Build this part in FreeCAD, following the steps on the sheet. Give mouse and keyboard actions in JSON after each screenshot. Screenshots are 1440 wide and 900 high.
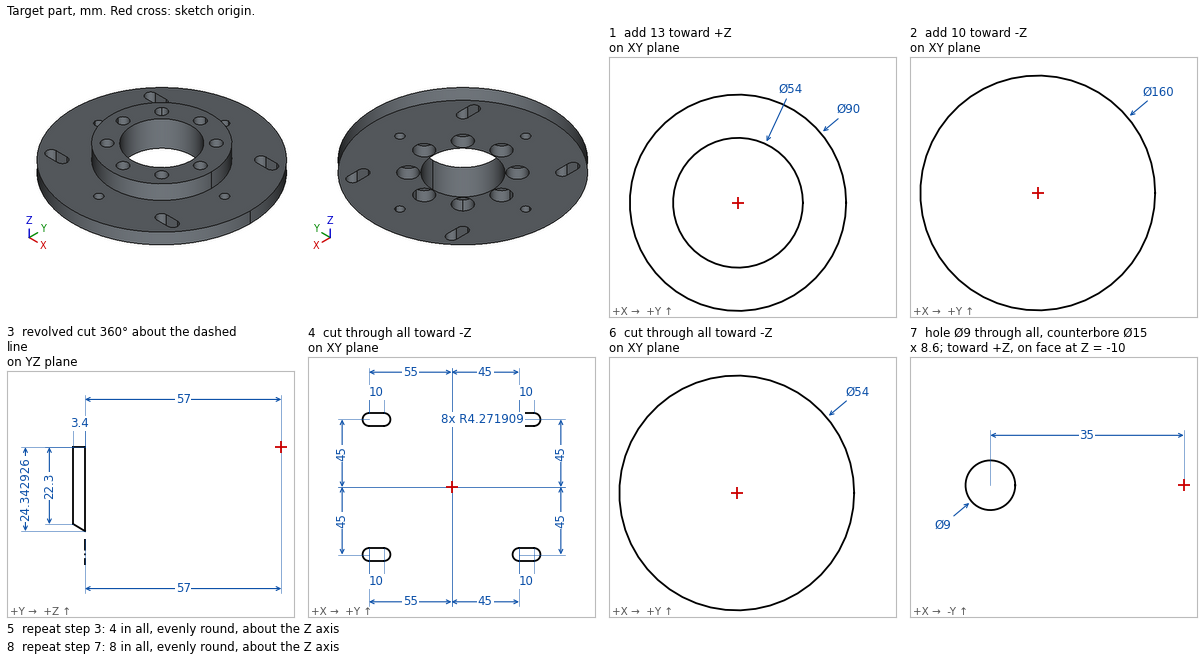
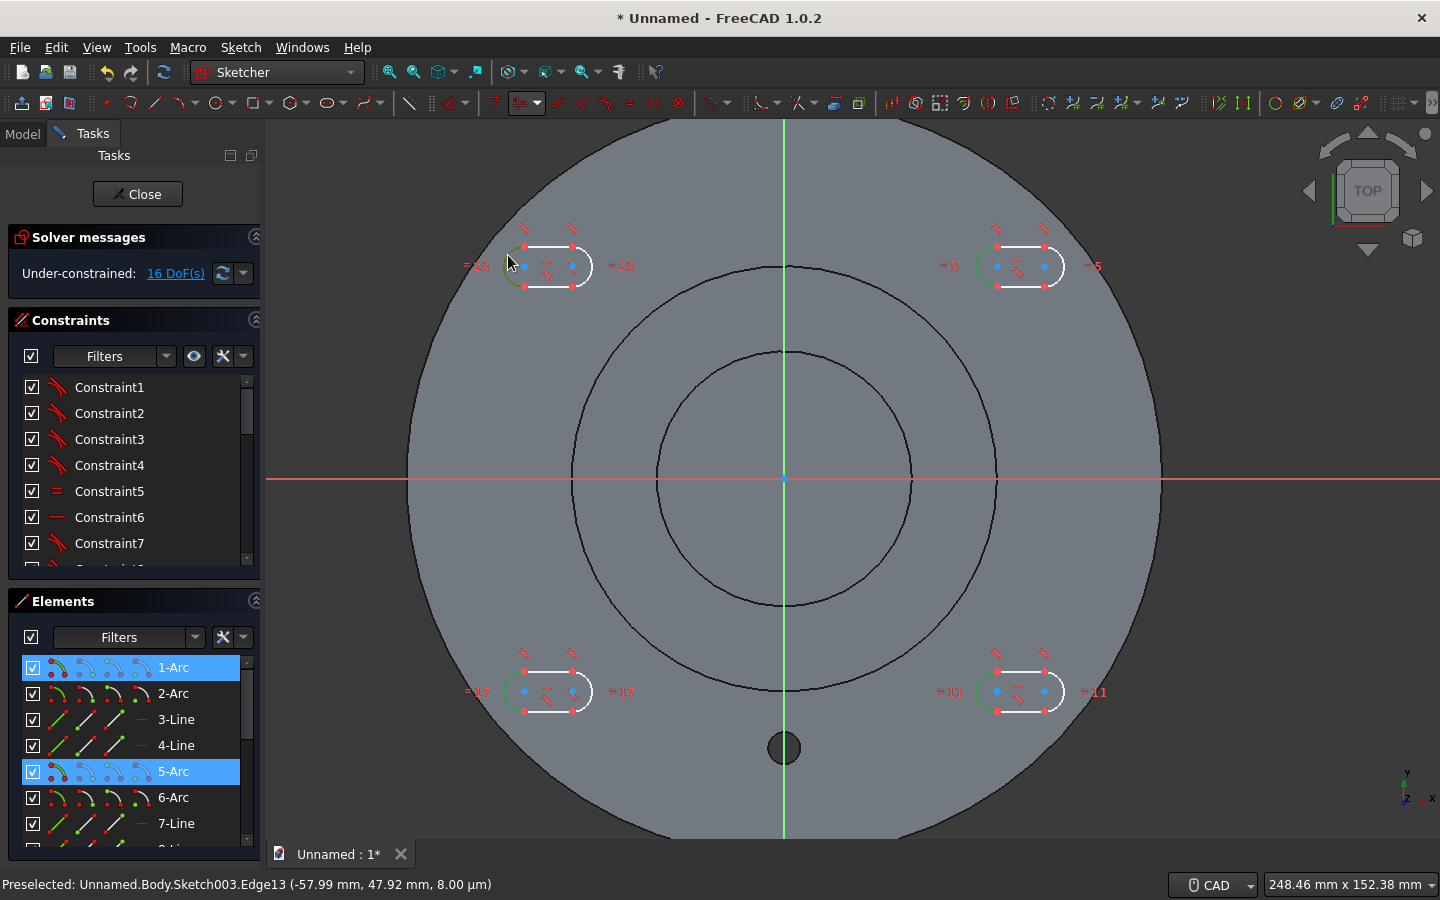
{"action": "key", "text": "e"}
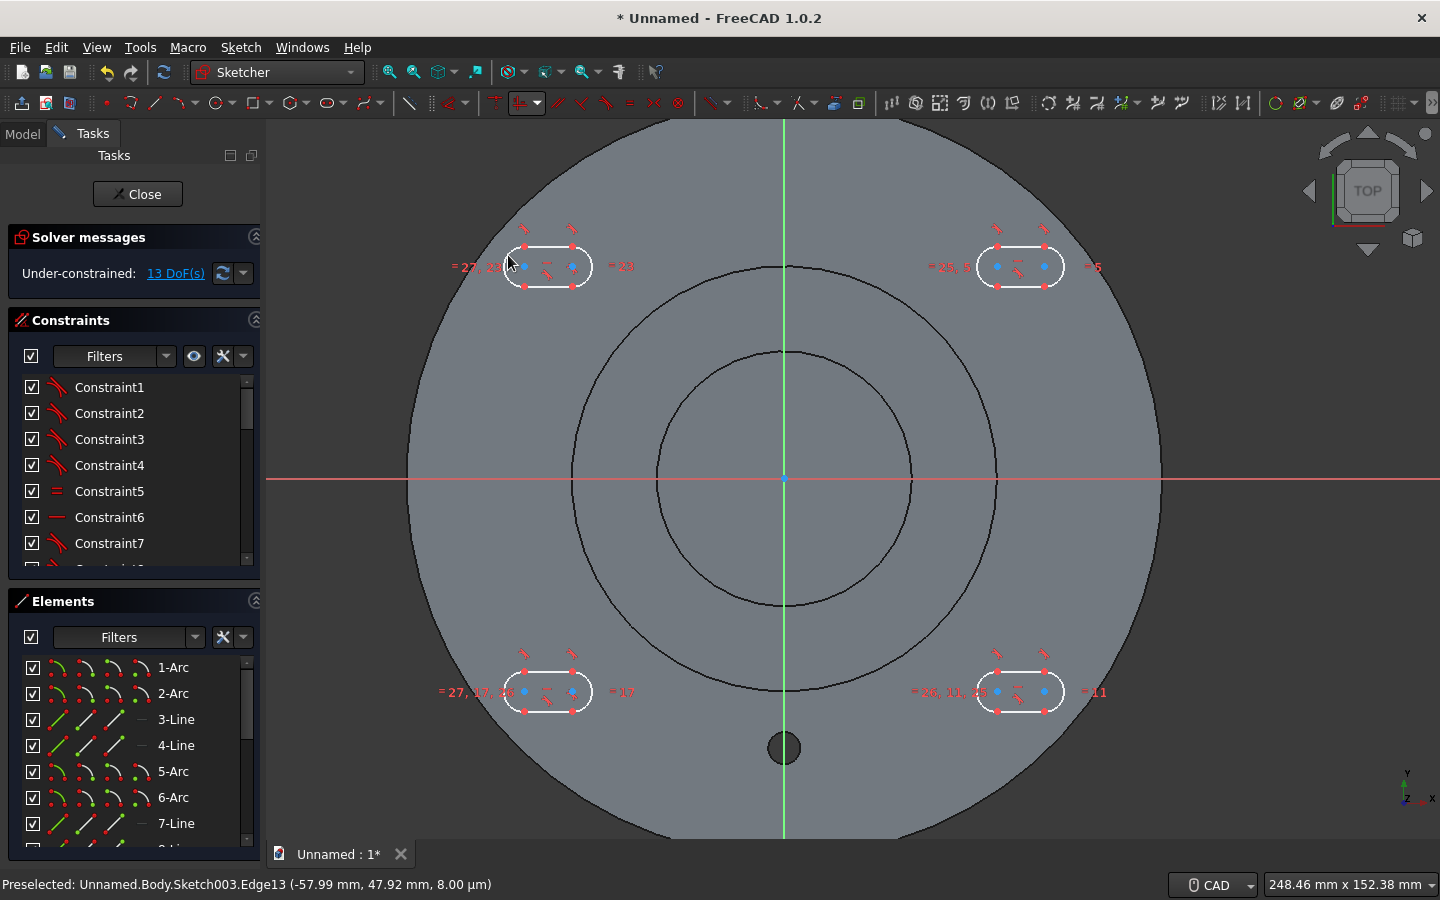
{"action": "key", "text": "d"}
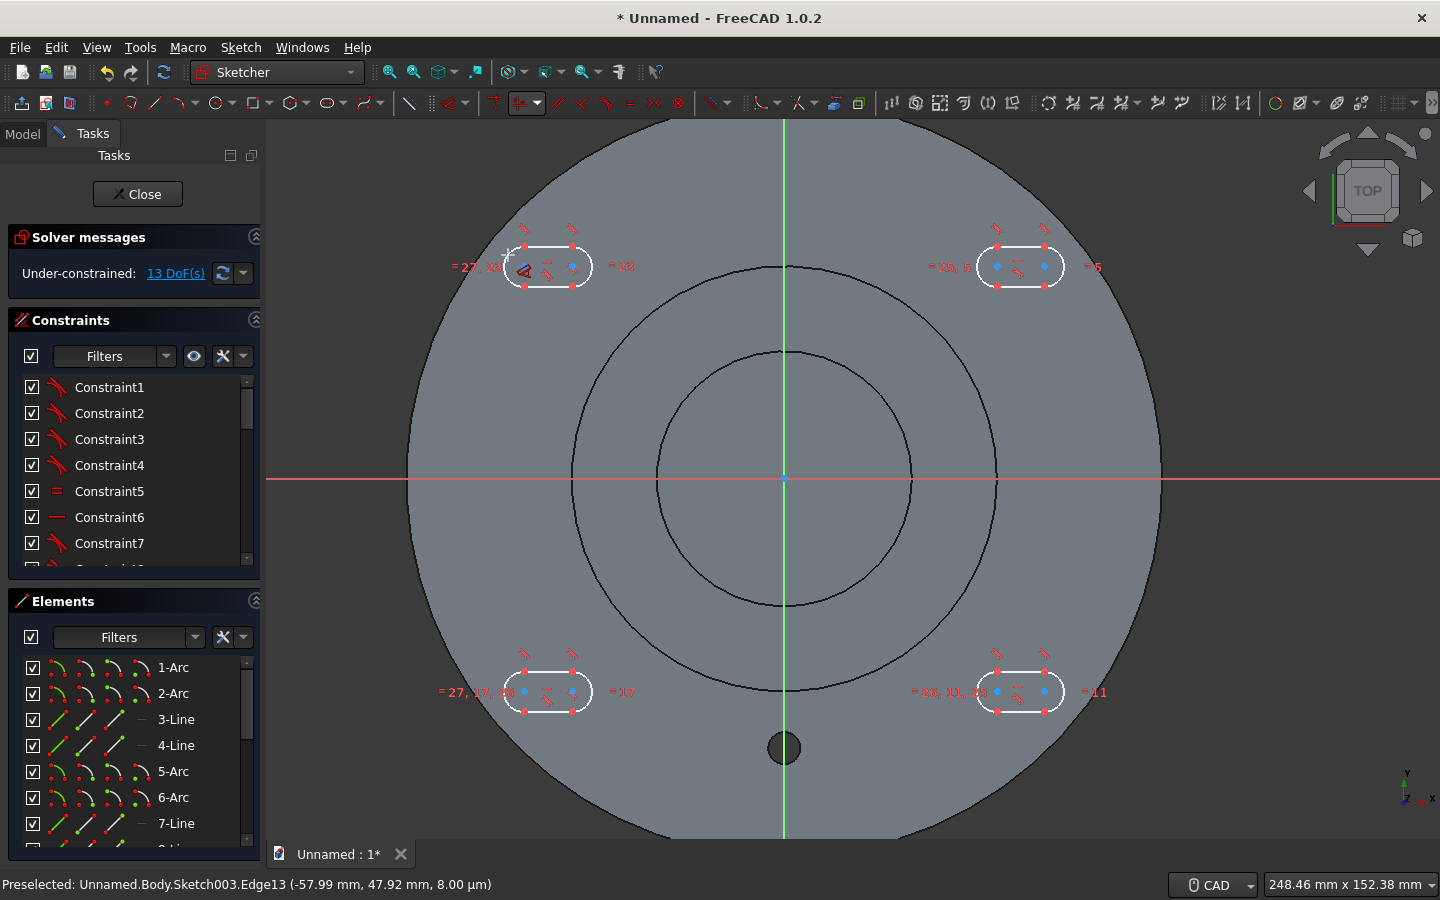
{"action": "scroll", "coordinate": [981, 255], "scroll_direction": "up", "scroll_amount": 4}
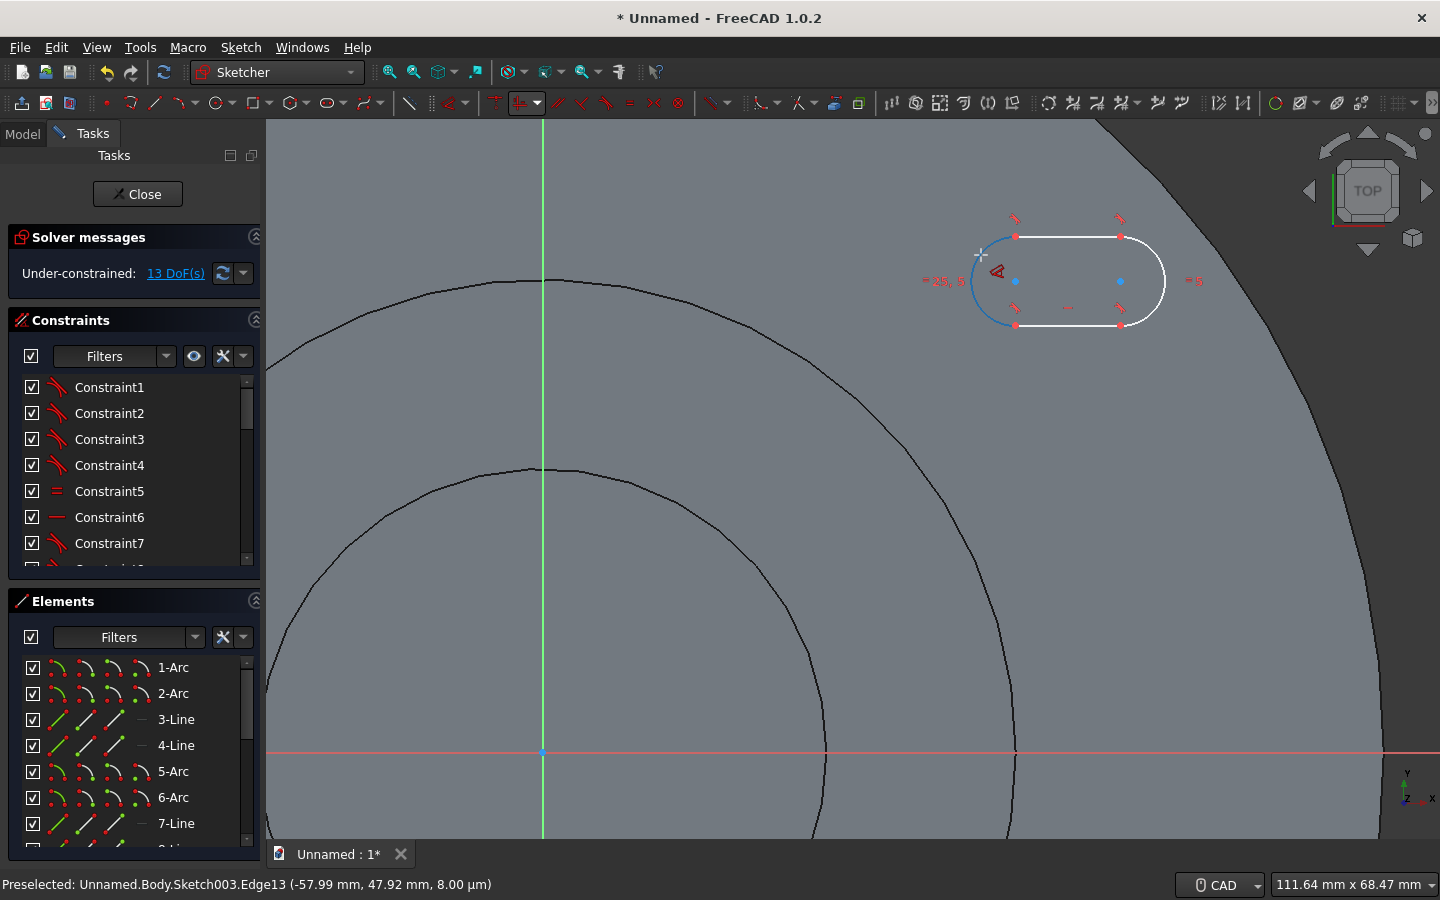
{"action": "left_click", "coordinate": [980, 255]}
{"action": "left_click", "coordinate": [954, 236]}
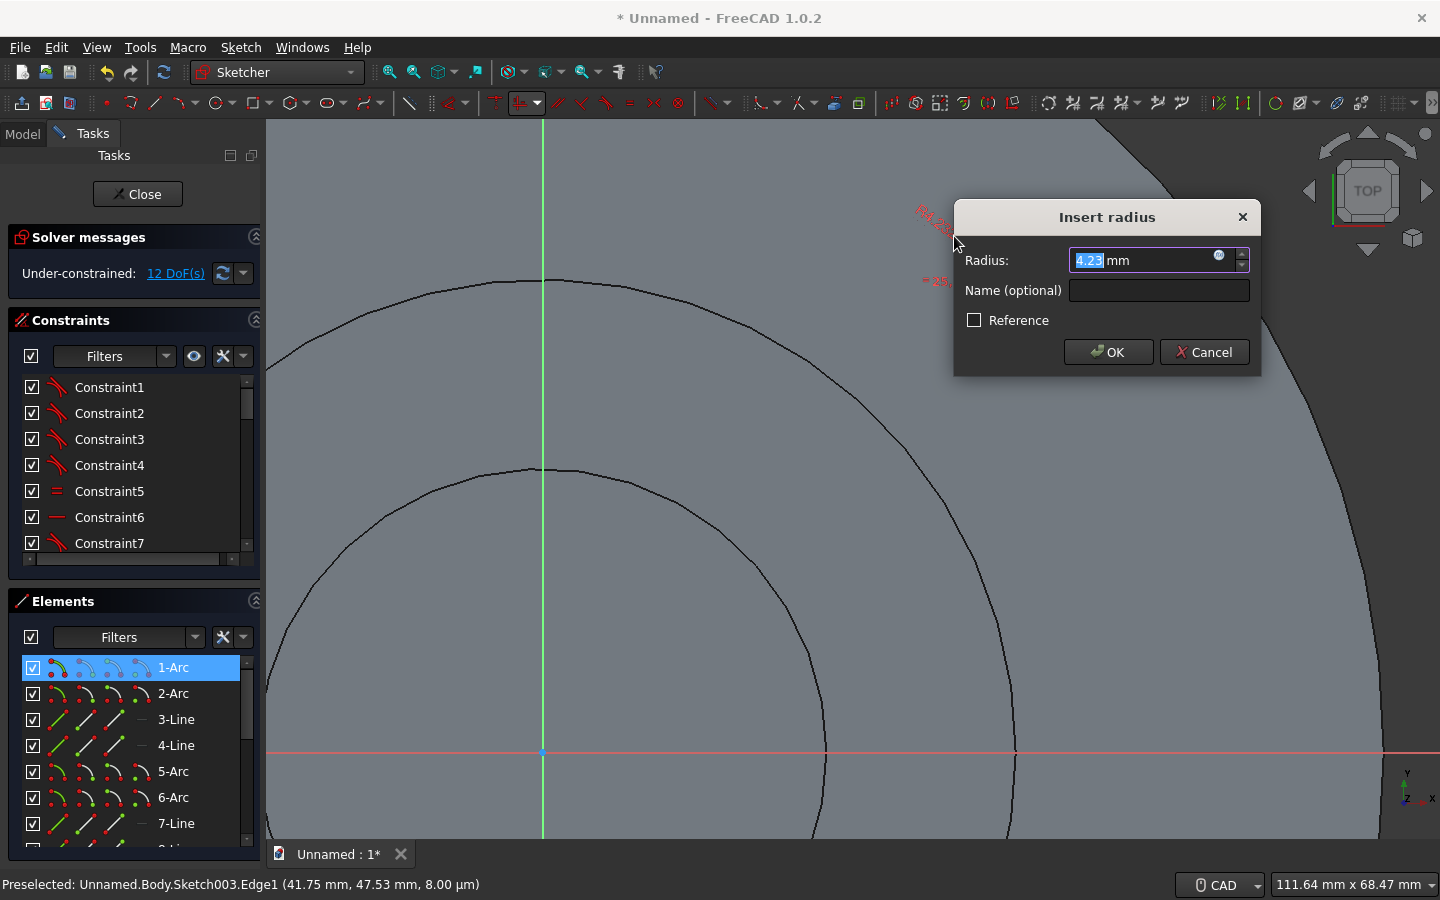
{"action": "type", "text": "4.271909"}
{"action": "key", "text": "Return"}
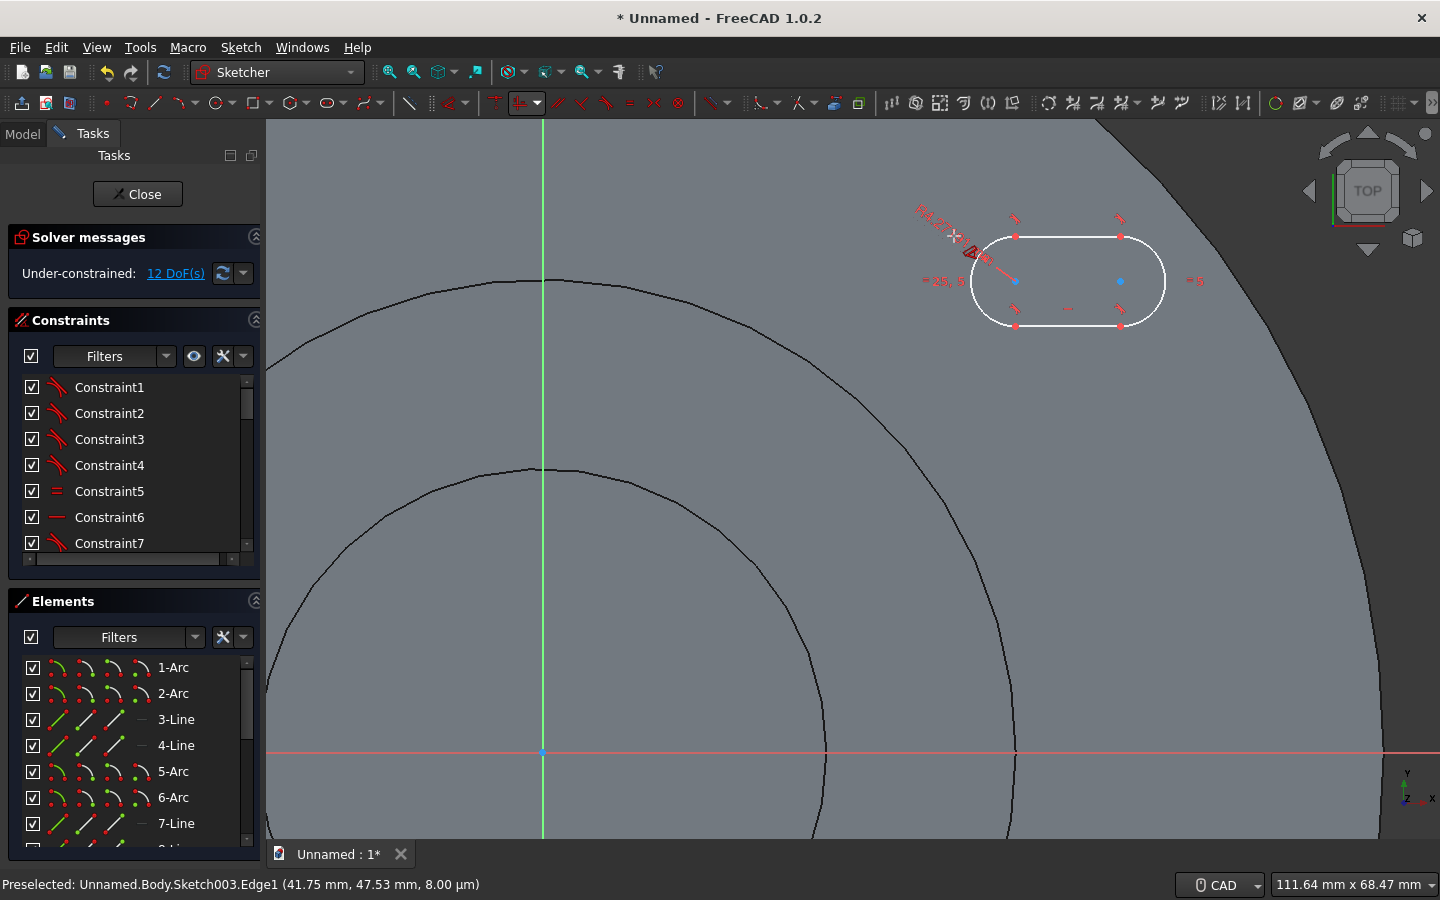
{"action": "left_click", "coordinate": [1047, 237]}
{"action": "left_click", "coordinate": [1068, 203]}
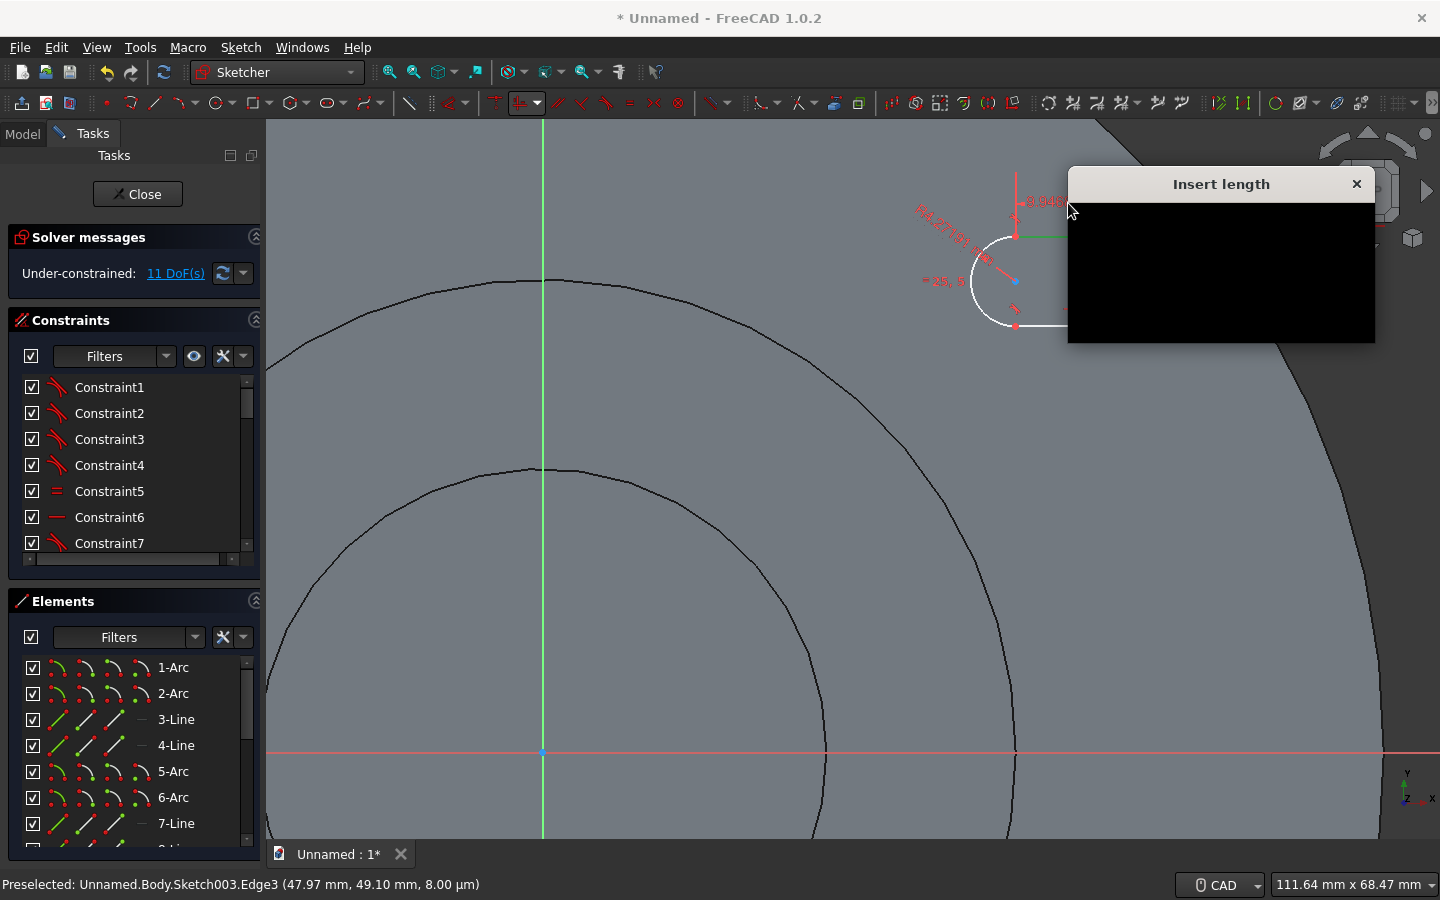
{"action": "type", "text": "10"}
{"action": "key", "text": "Return"}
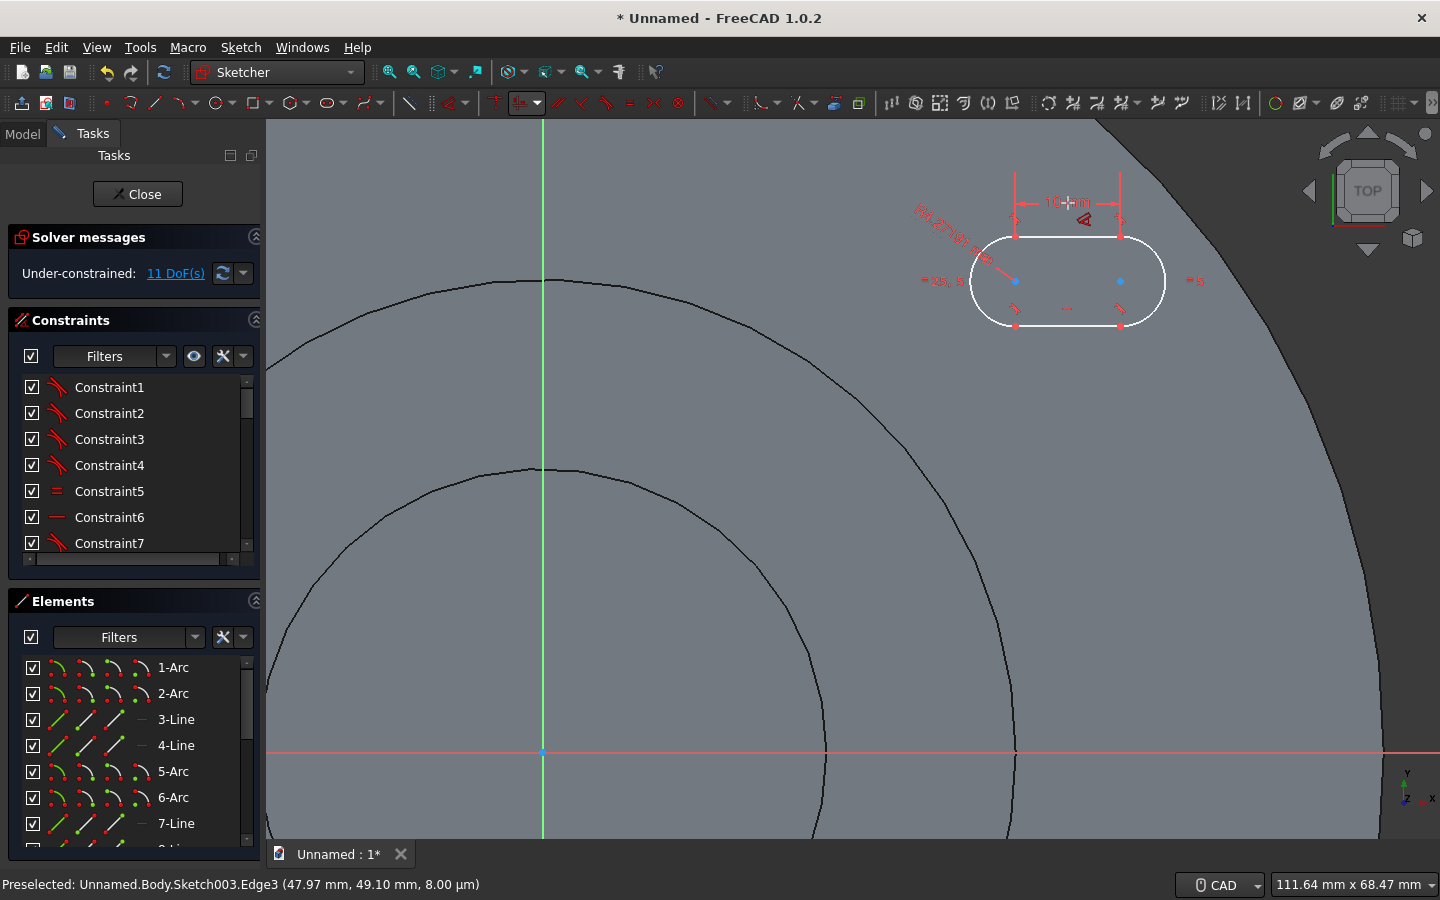
{"action": "scroll", "coordinate": [982, 255], "scroll_direction": "down", "scroll_amount": 4}